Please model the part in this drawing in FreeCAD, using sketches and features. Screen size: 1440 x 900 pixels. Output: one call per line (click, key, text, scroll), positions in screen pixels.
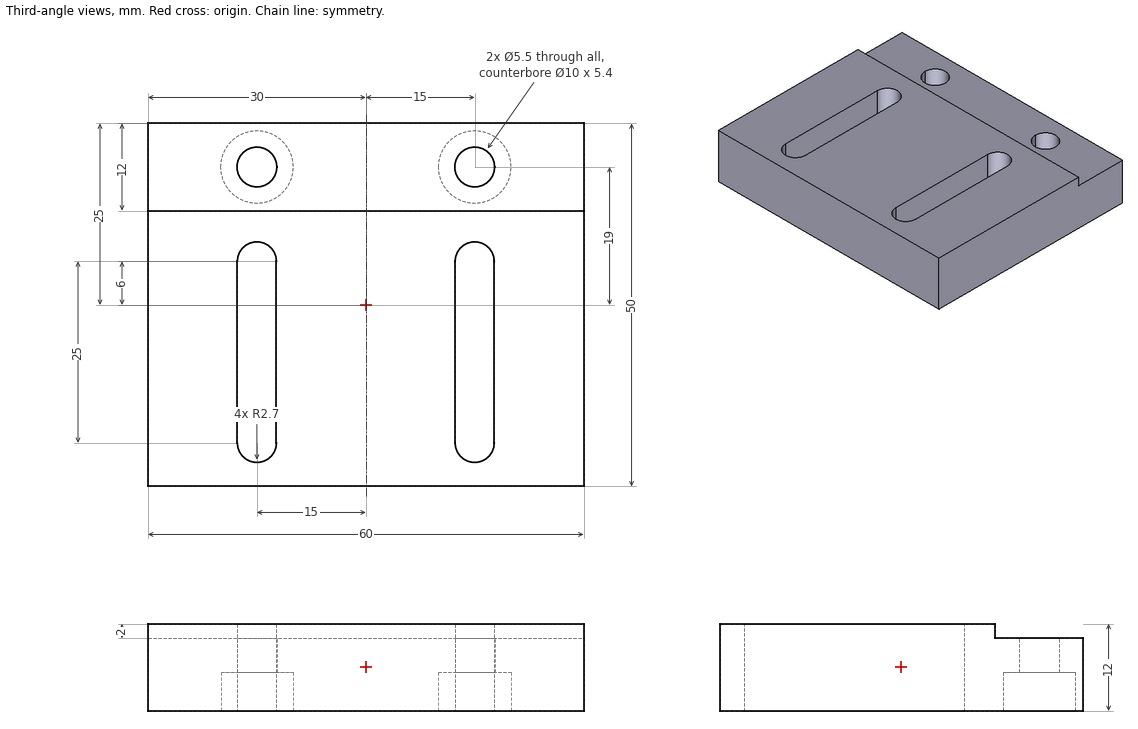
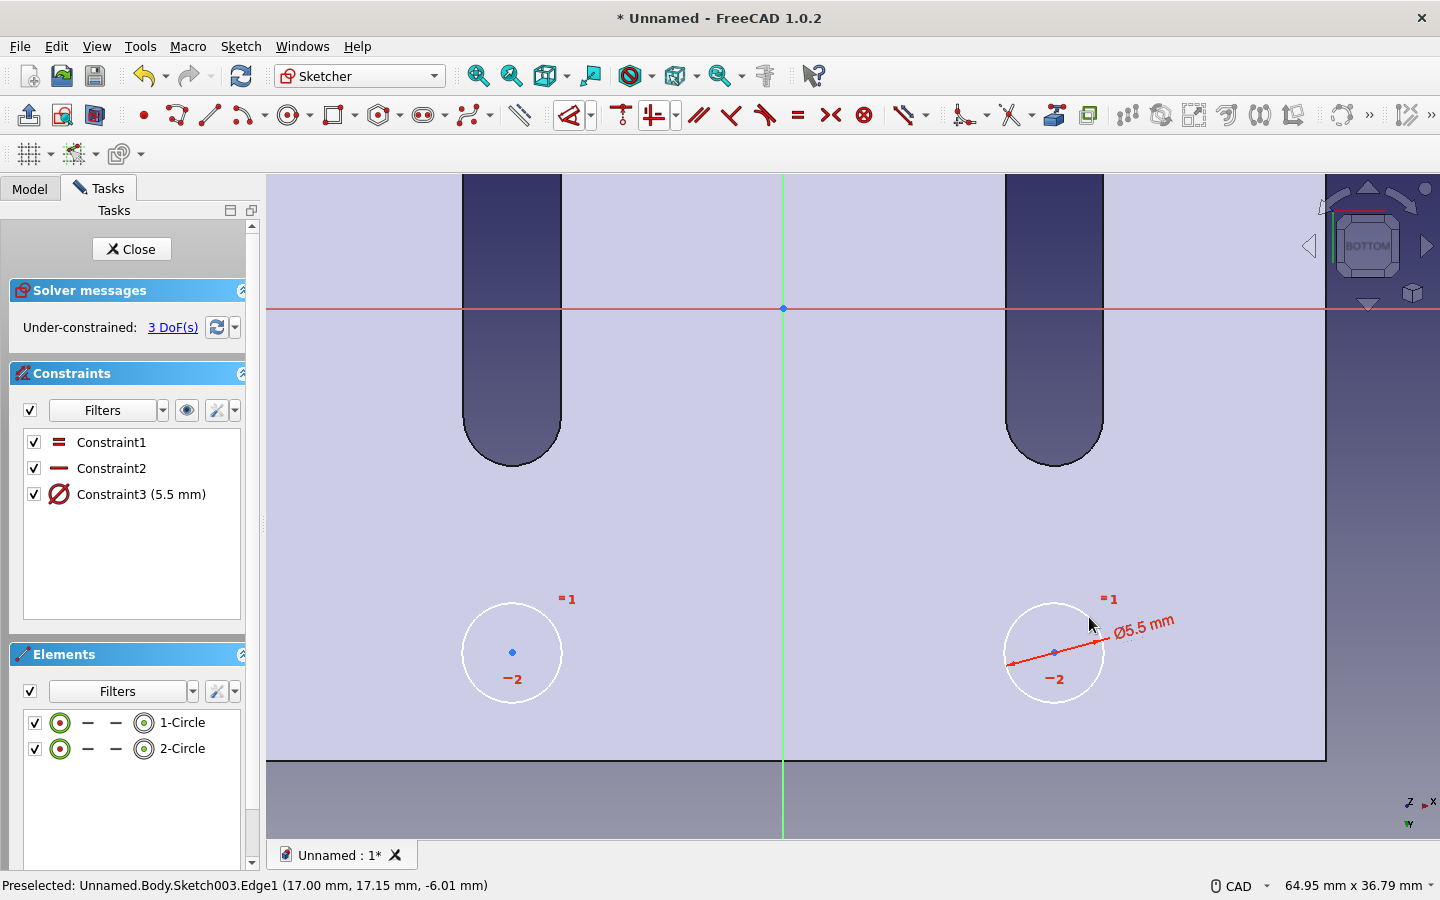
click(1054, 653)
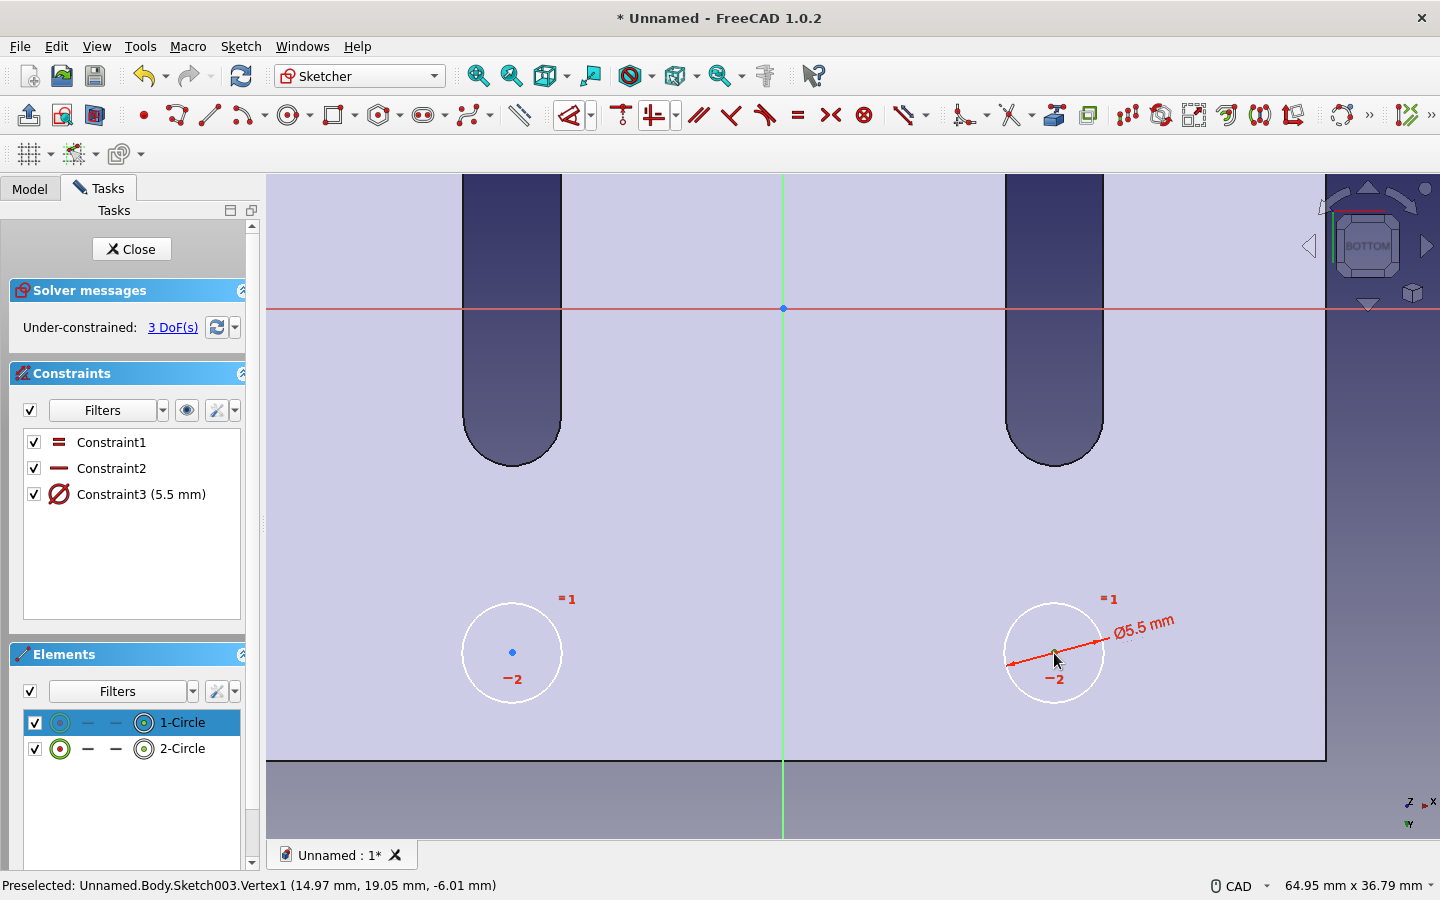
click(590, 116)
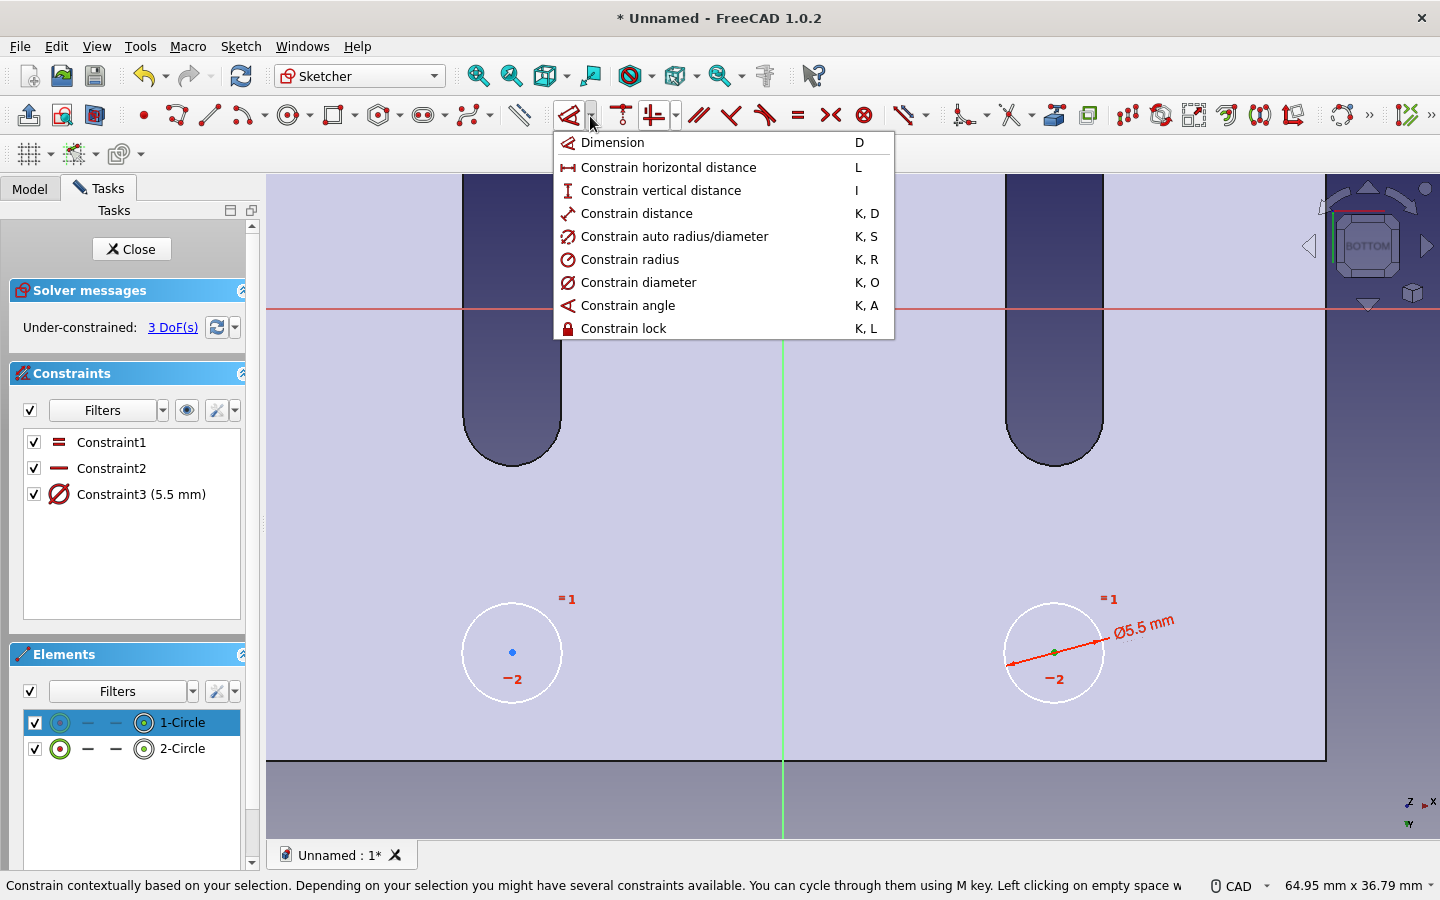
click(724, 168)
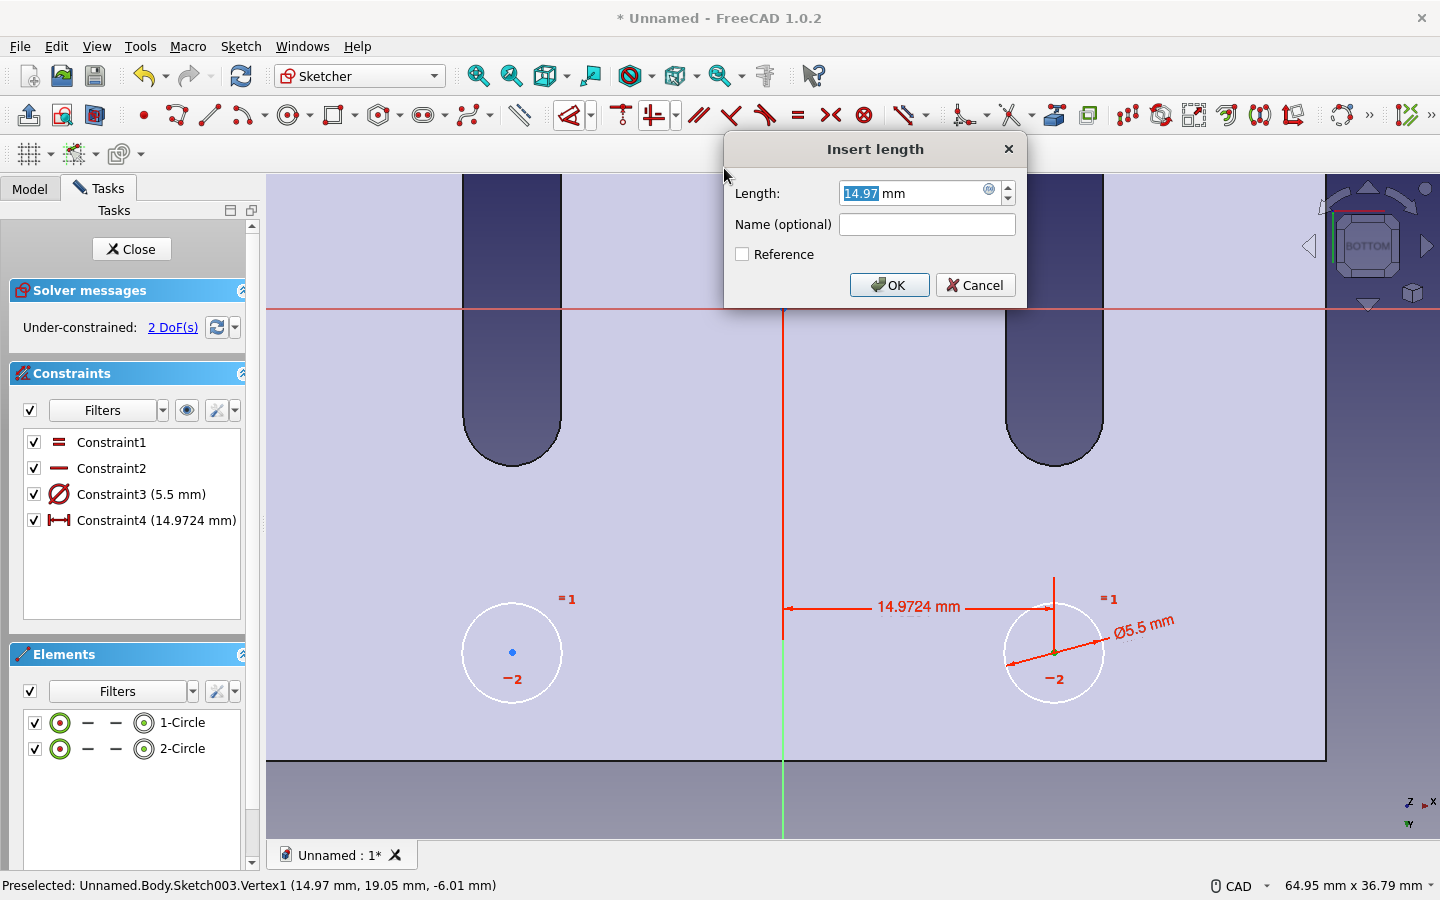
text(15)
key(Return)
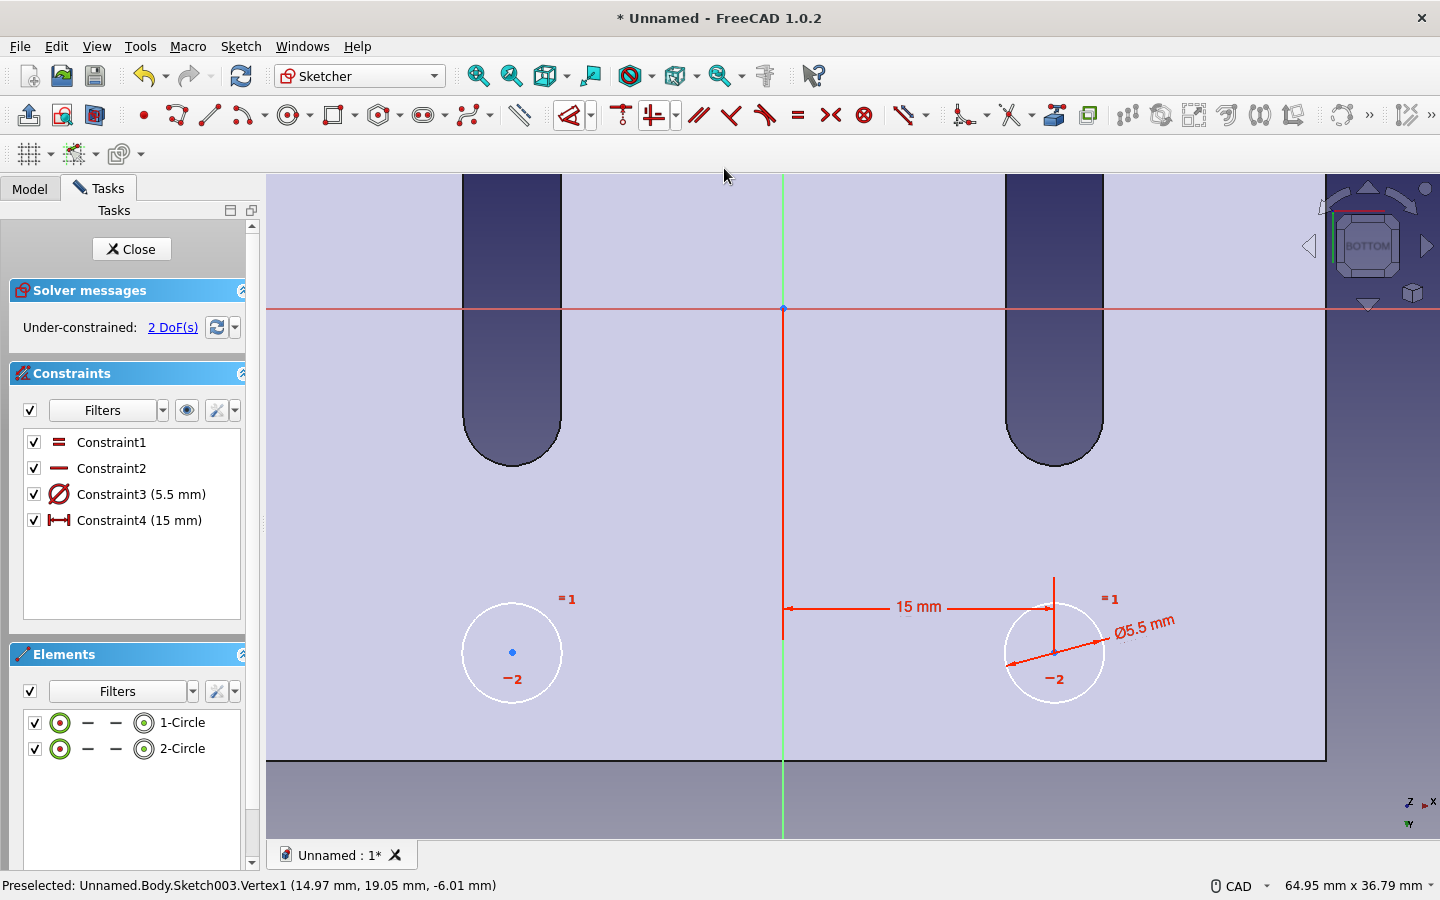
click(1054, 653)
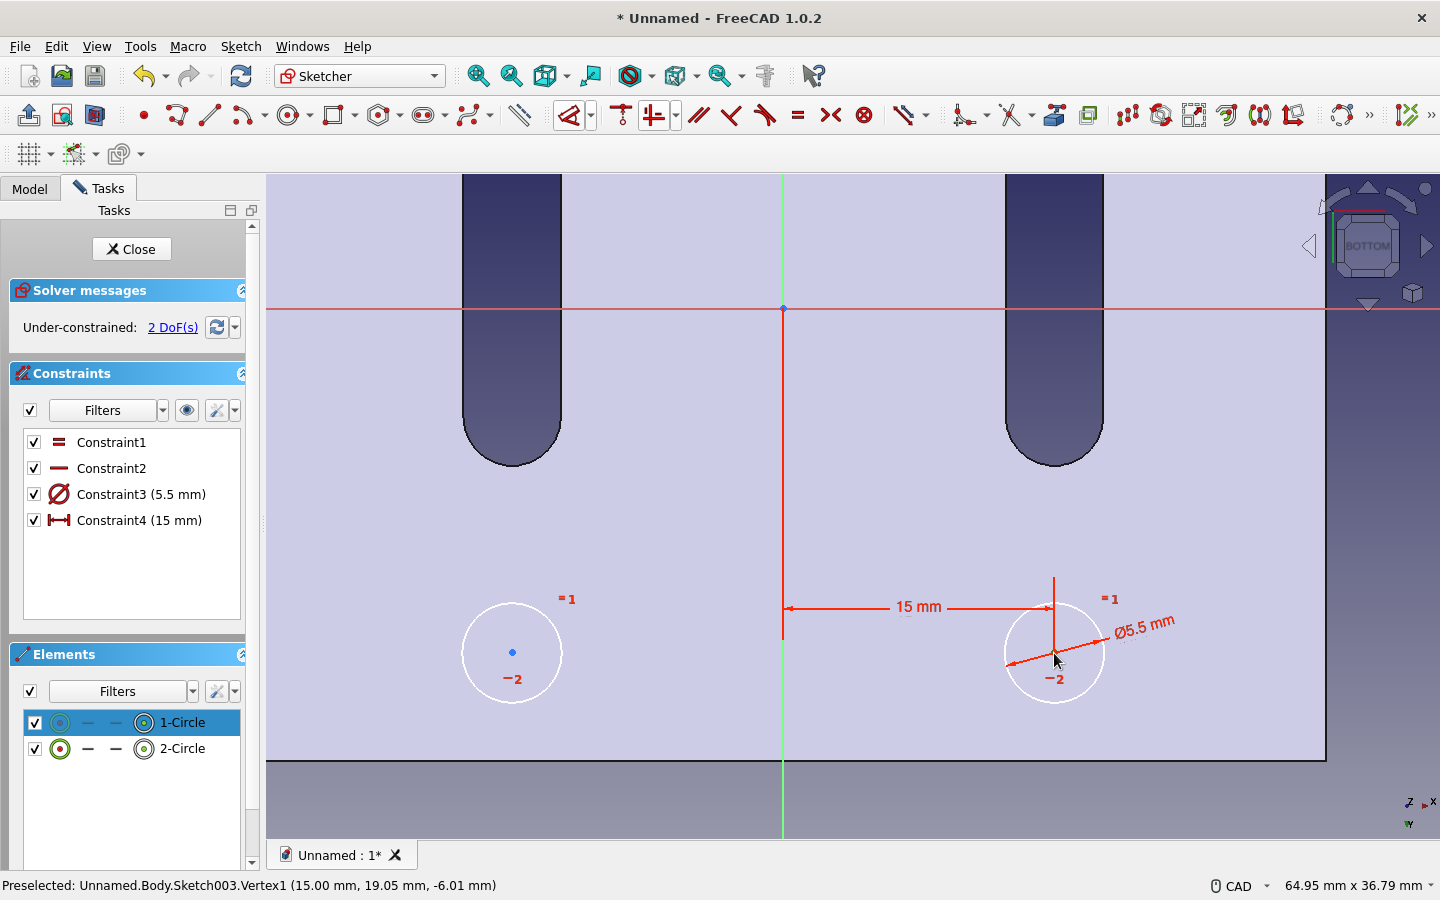
key(i)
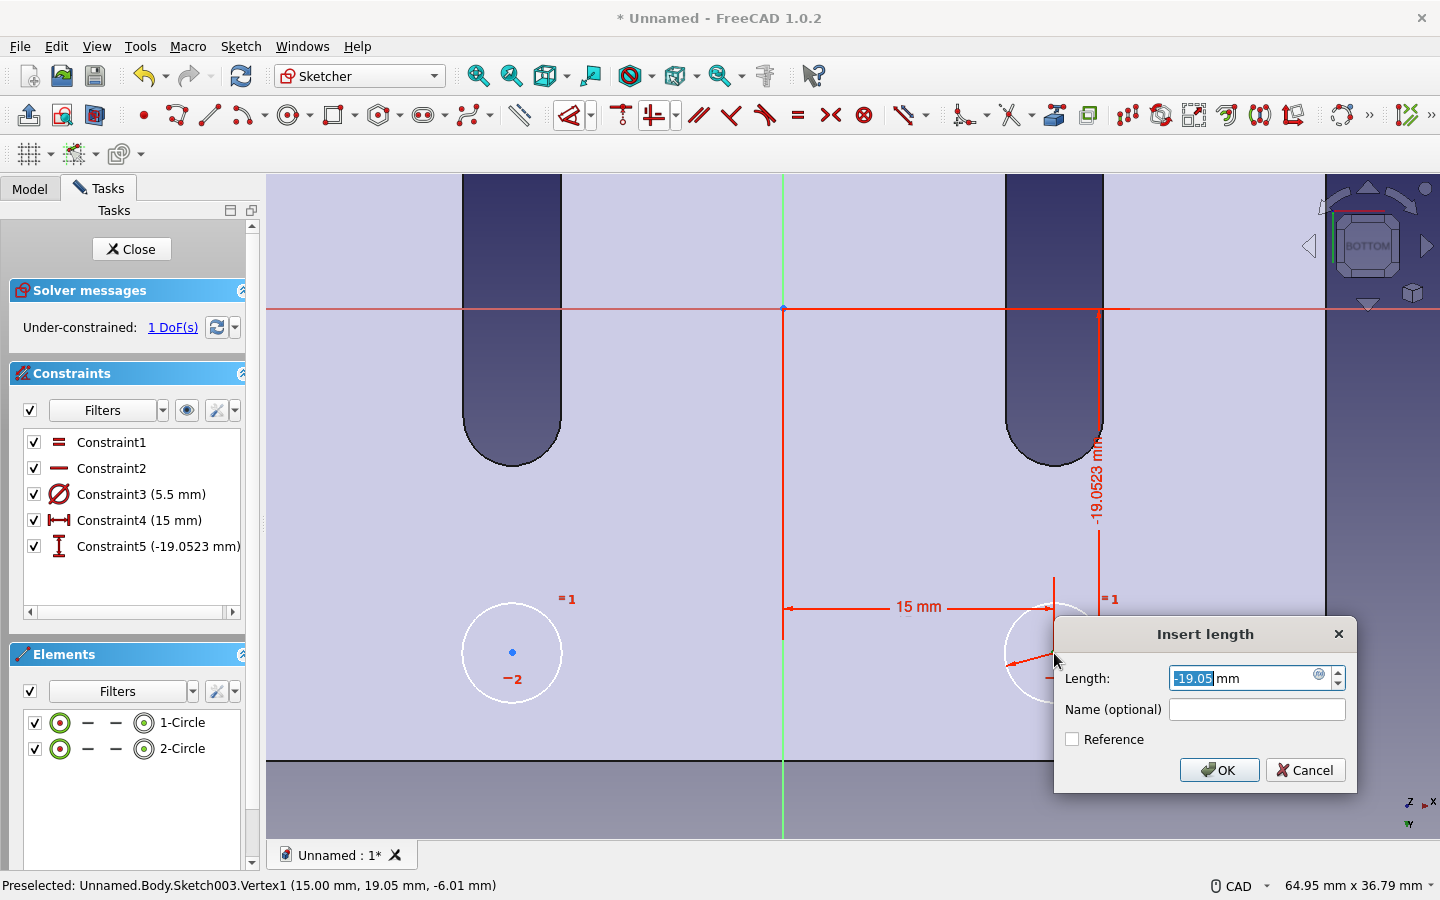
text(-19)
key(Return)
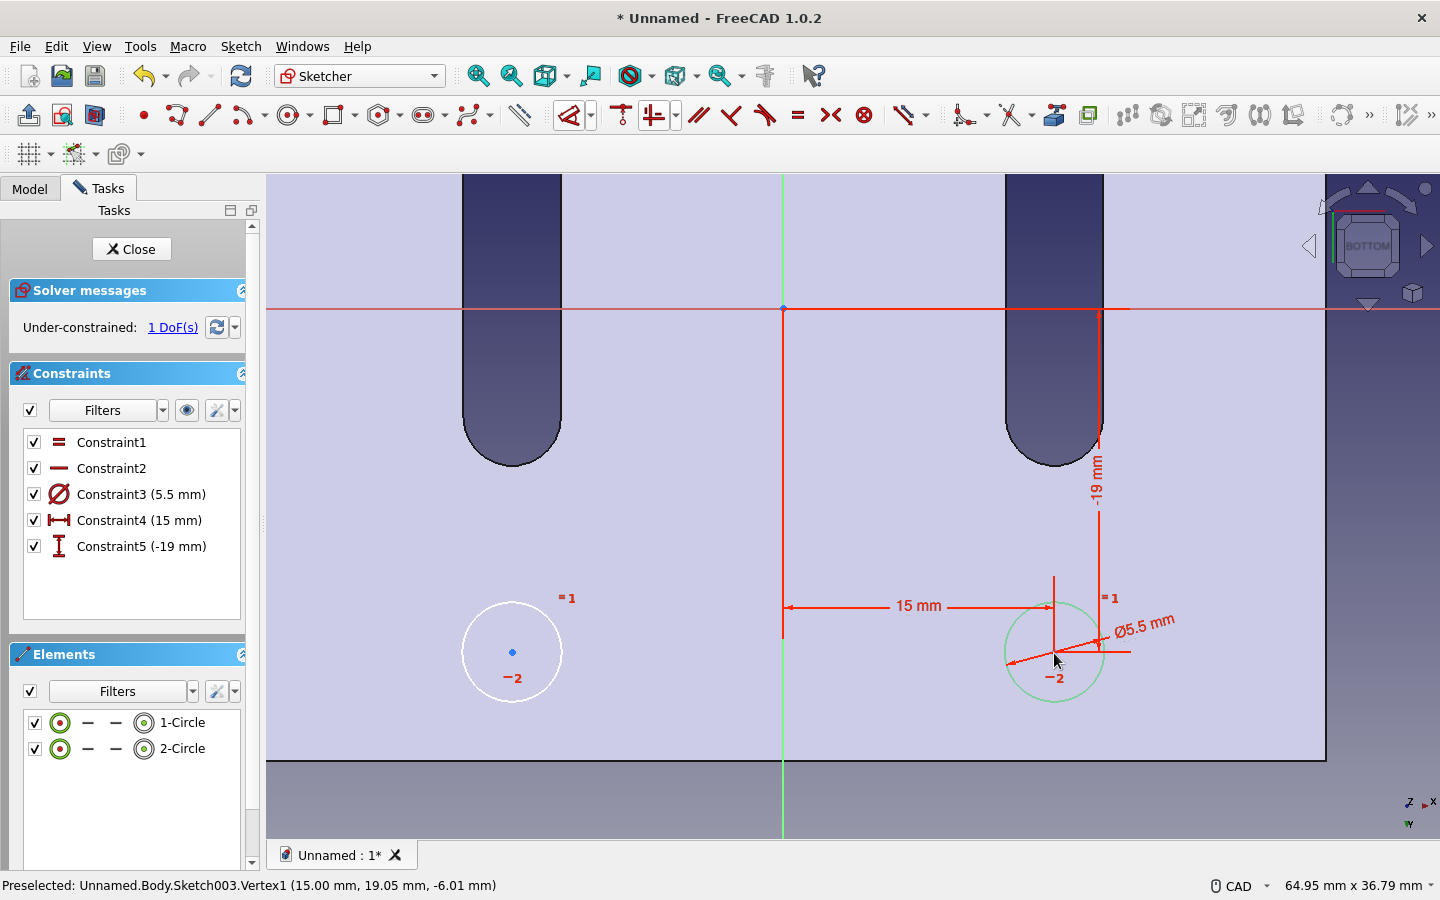
click(512, 652)